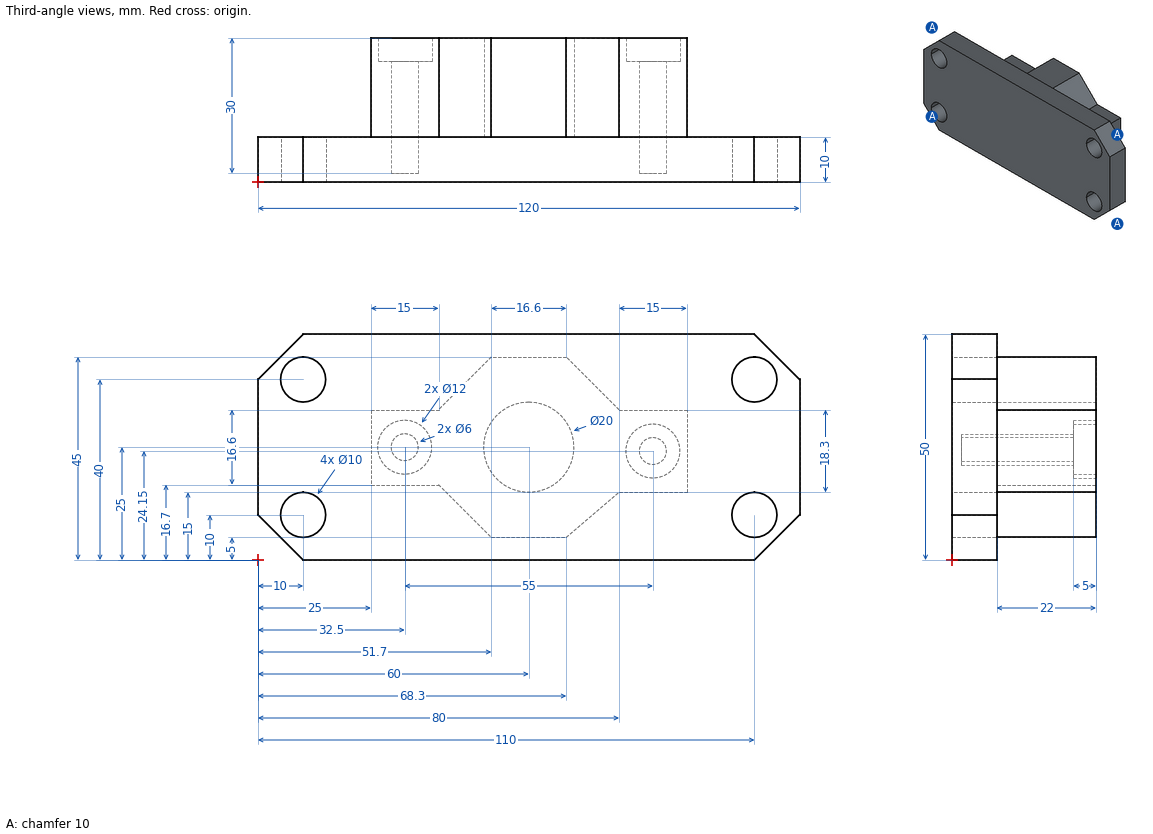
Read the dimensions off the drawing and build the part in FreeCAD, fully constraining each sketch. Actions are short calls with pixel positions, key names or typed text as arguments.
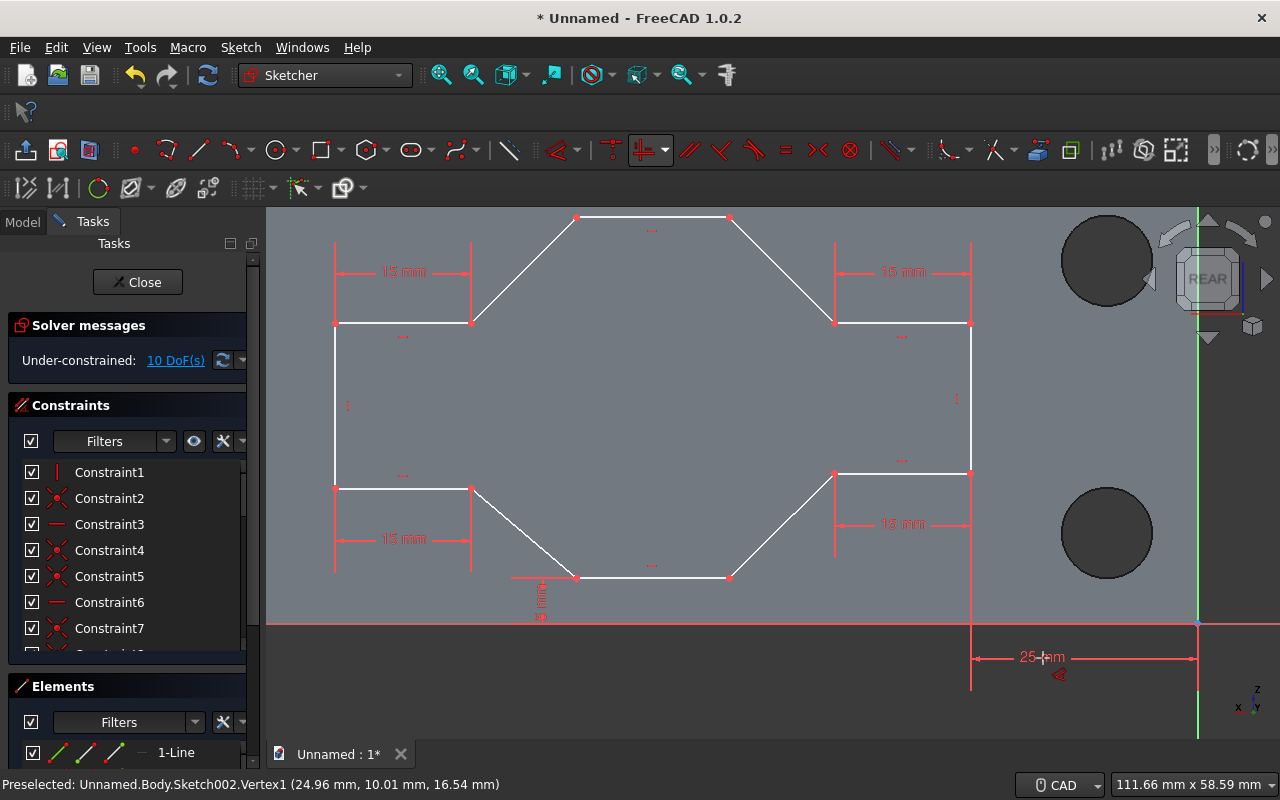
scroll(579, 582, down, 2)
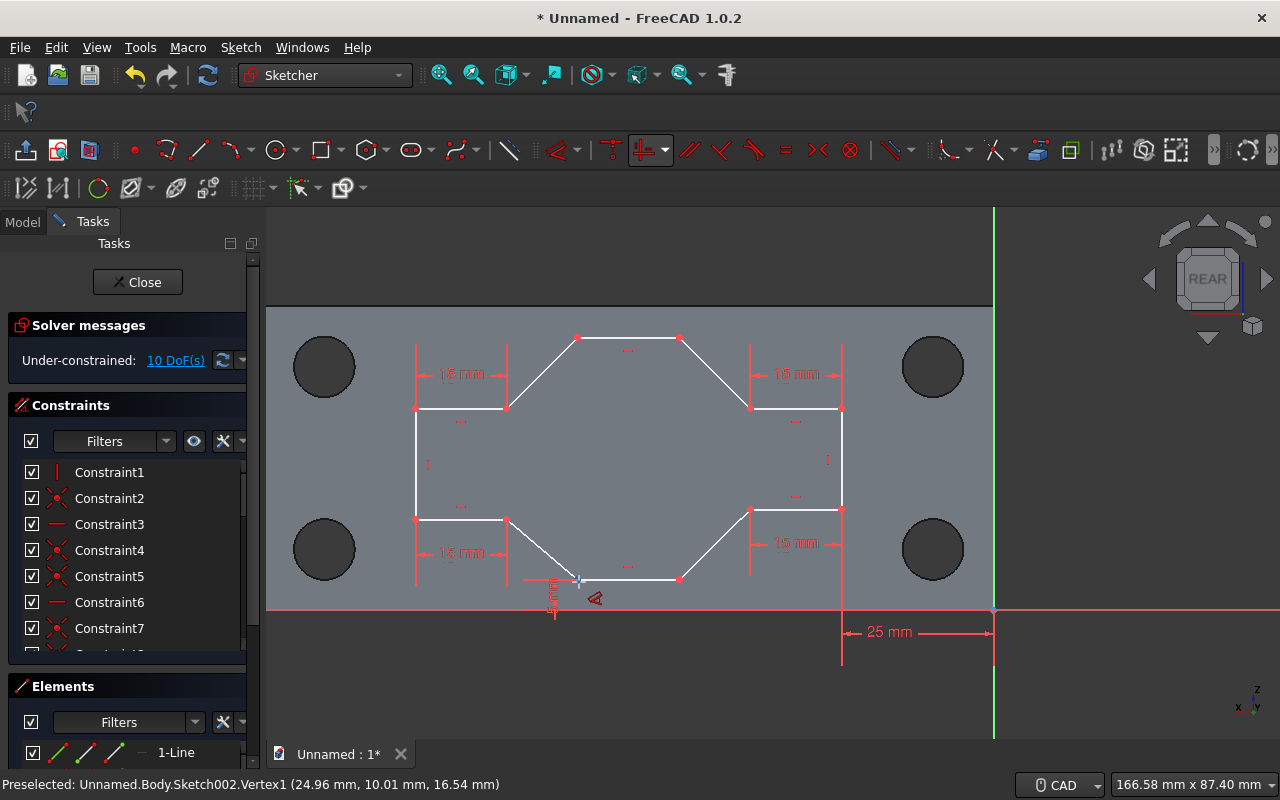
click(680, 338)
click(1028, 474)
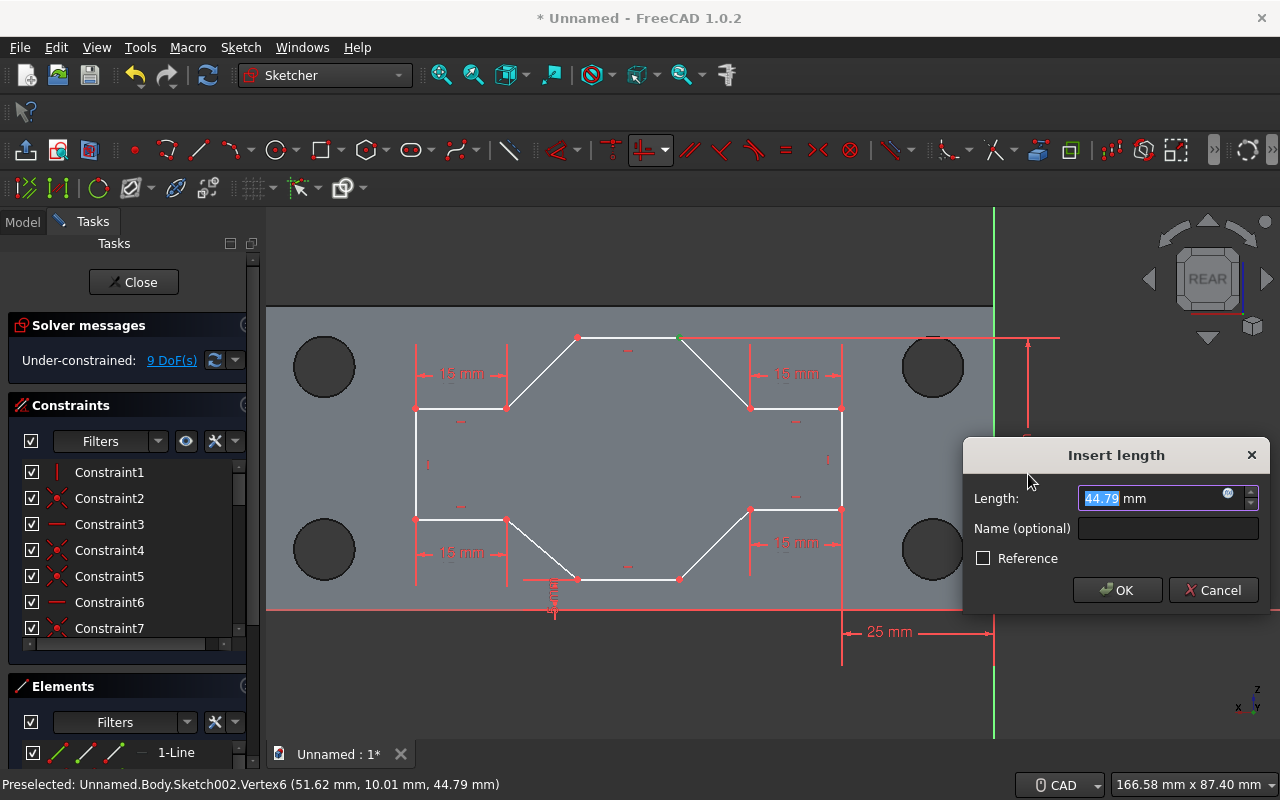
text(45)
key(Return)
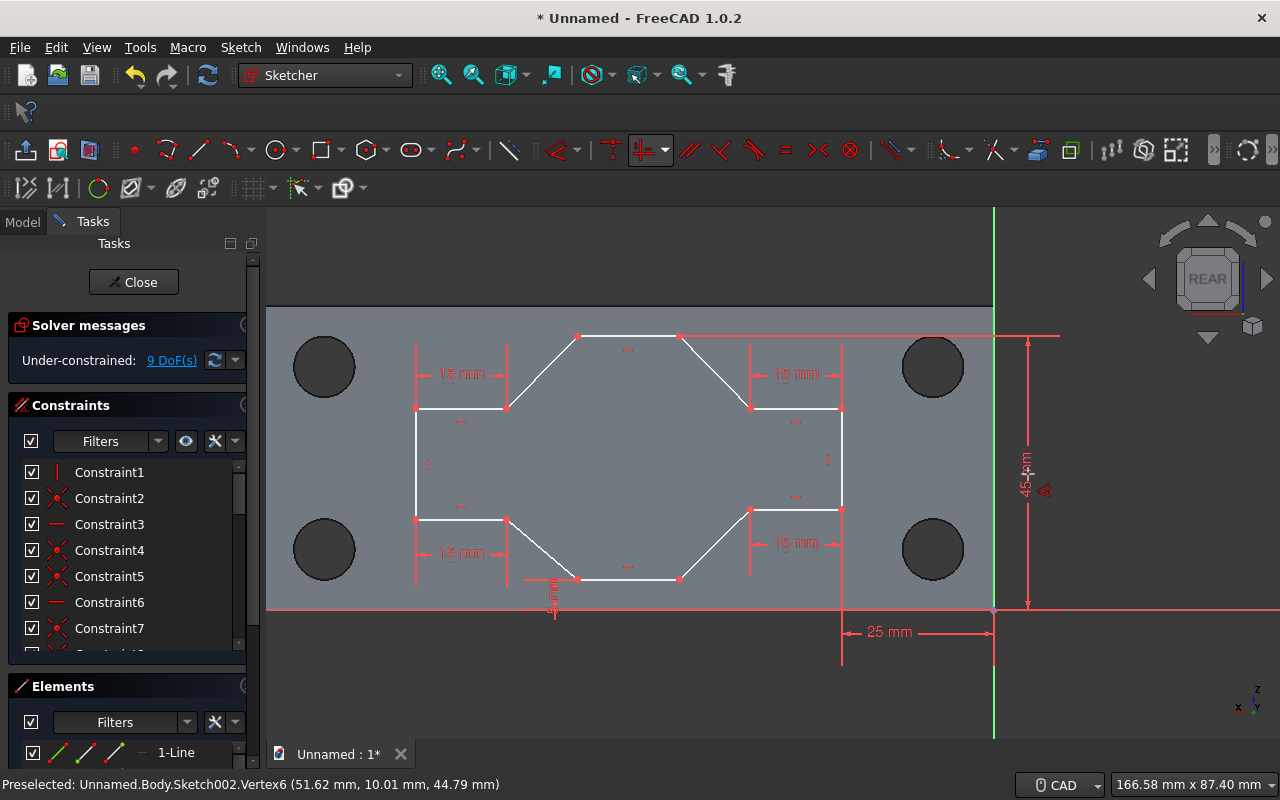
click(507, 409)
click(750, 644)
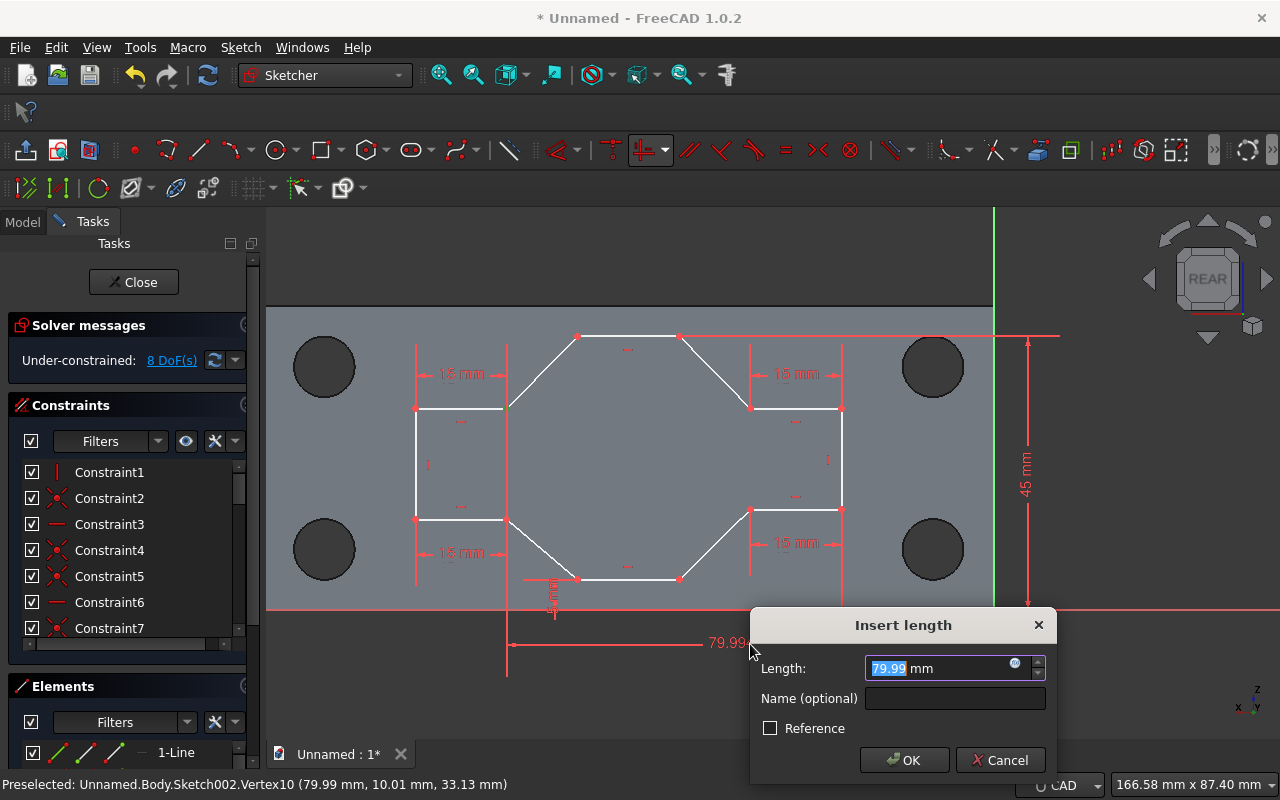
text(80)
key(Return)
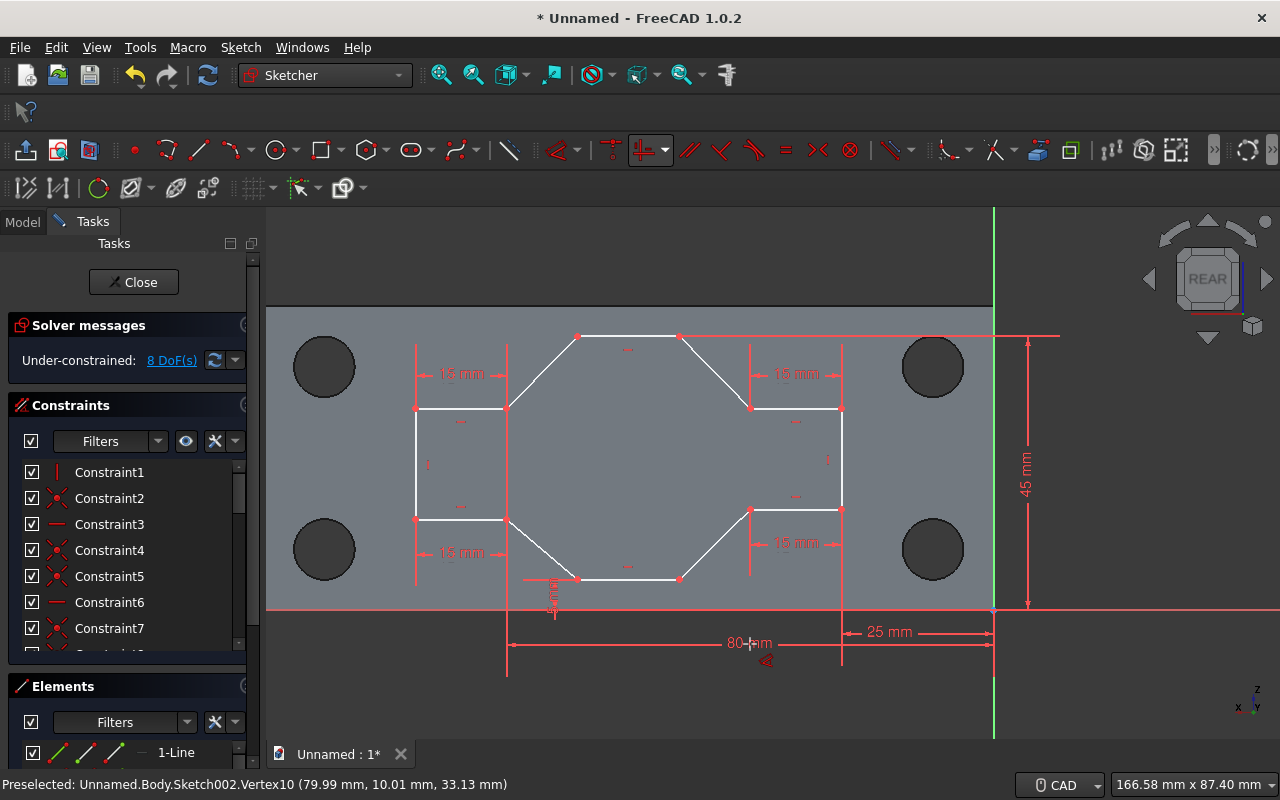
click(416, 520)
click(1028, 565)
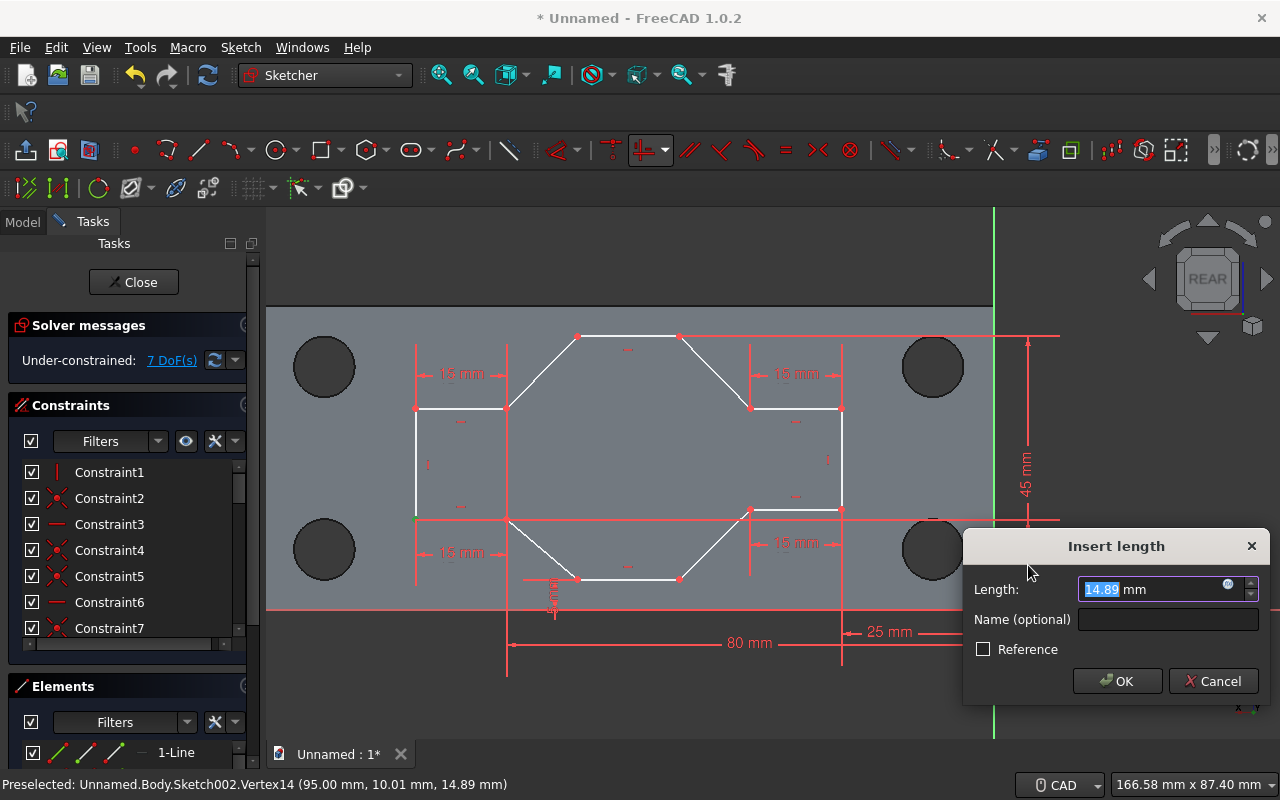
text(15)
key(Return)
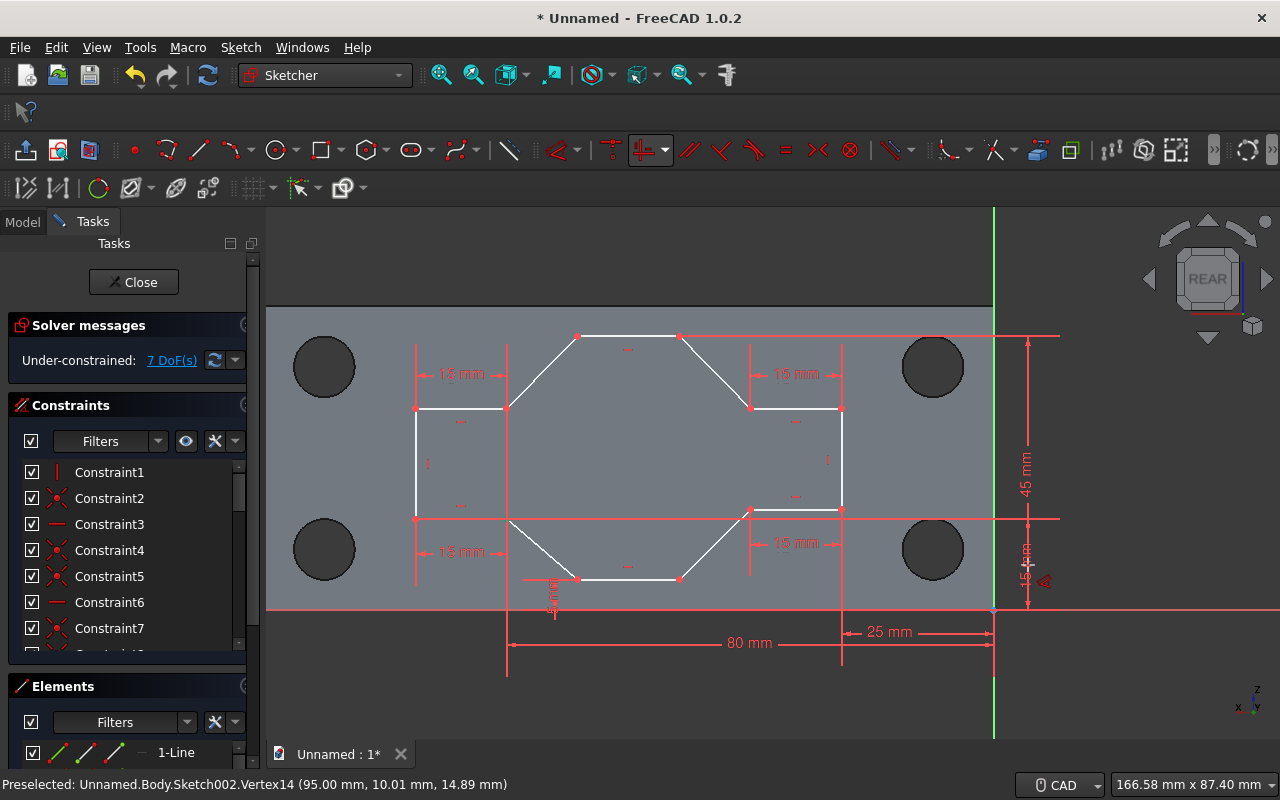
click(842, 479)
click(876, 459)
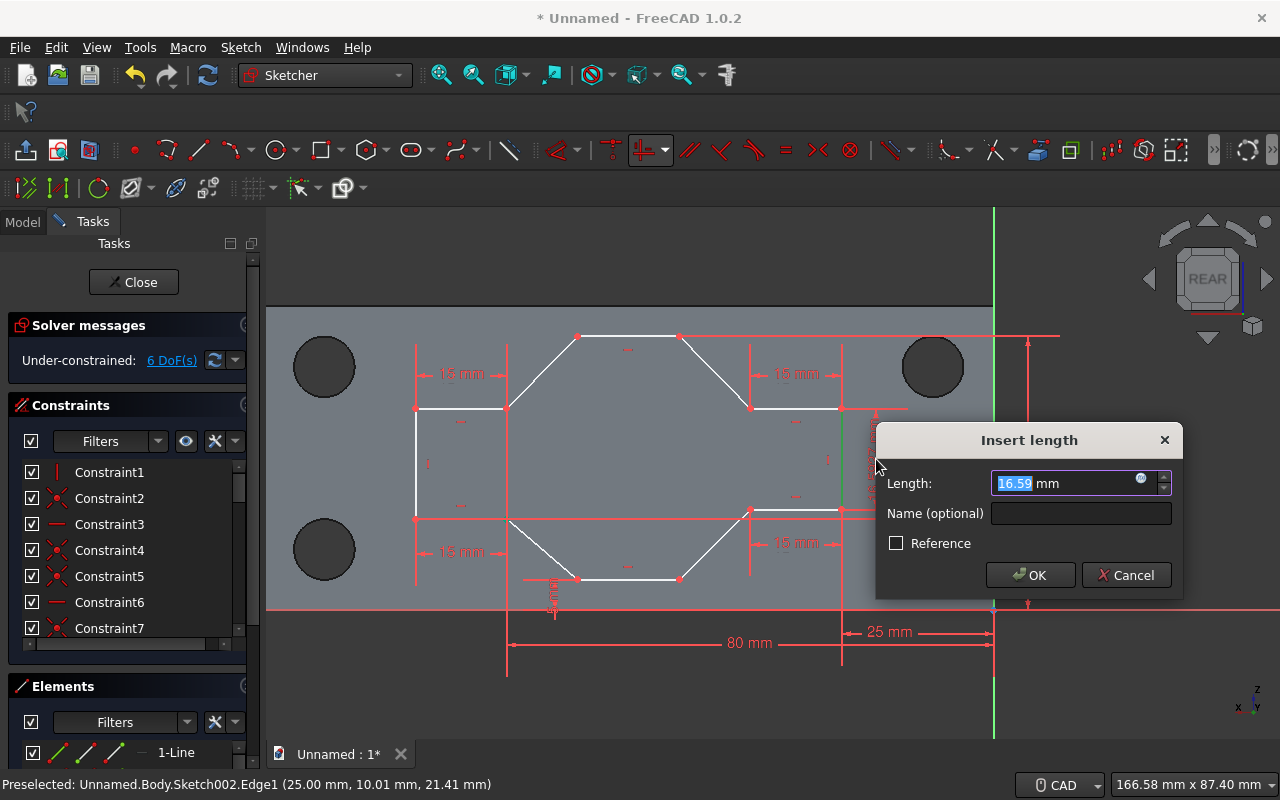
text(16.6)
key(Return)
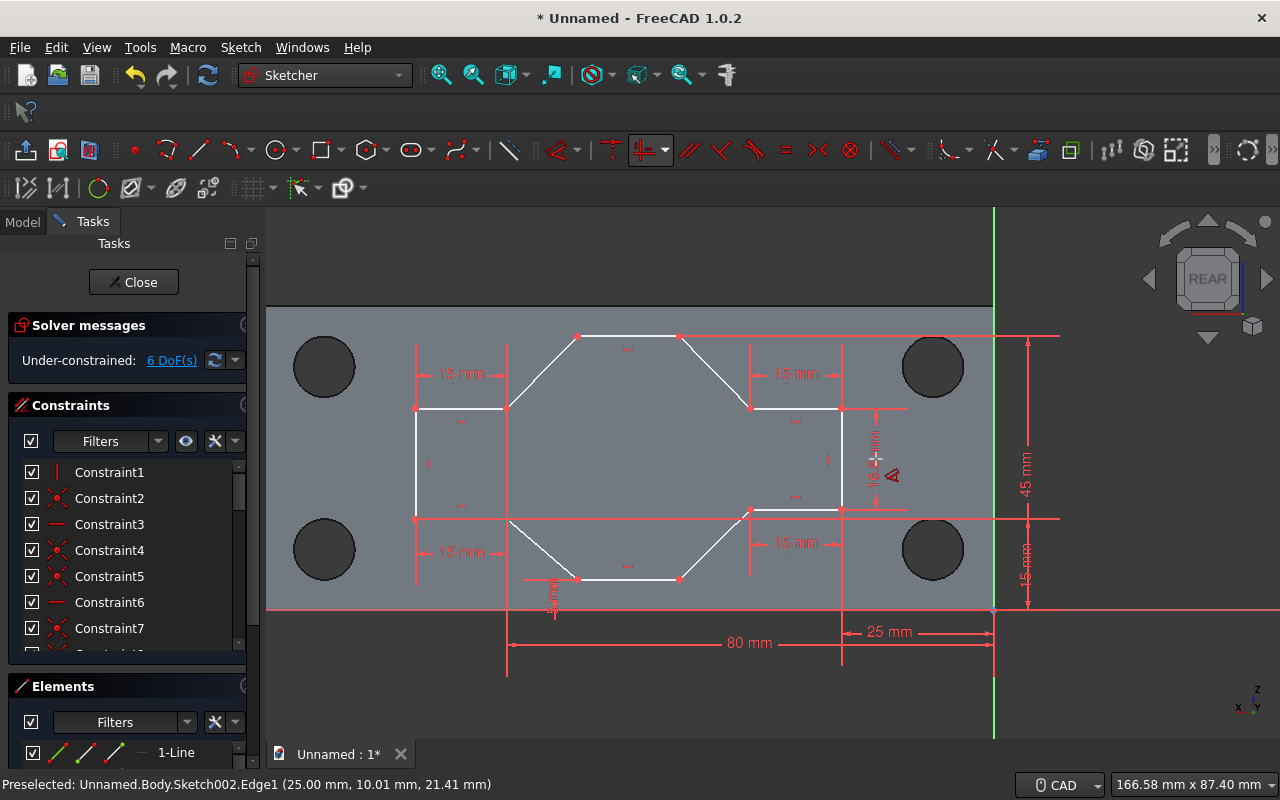
click(649, 336)
click(629, 302)